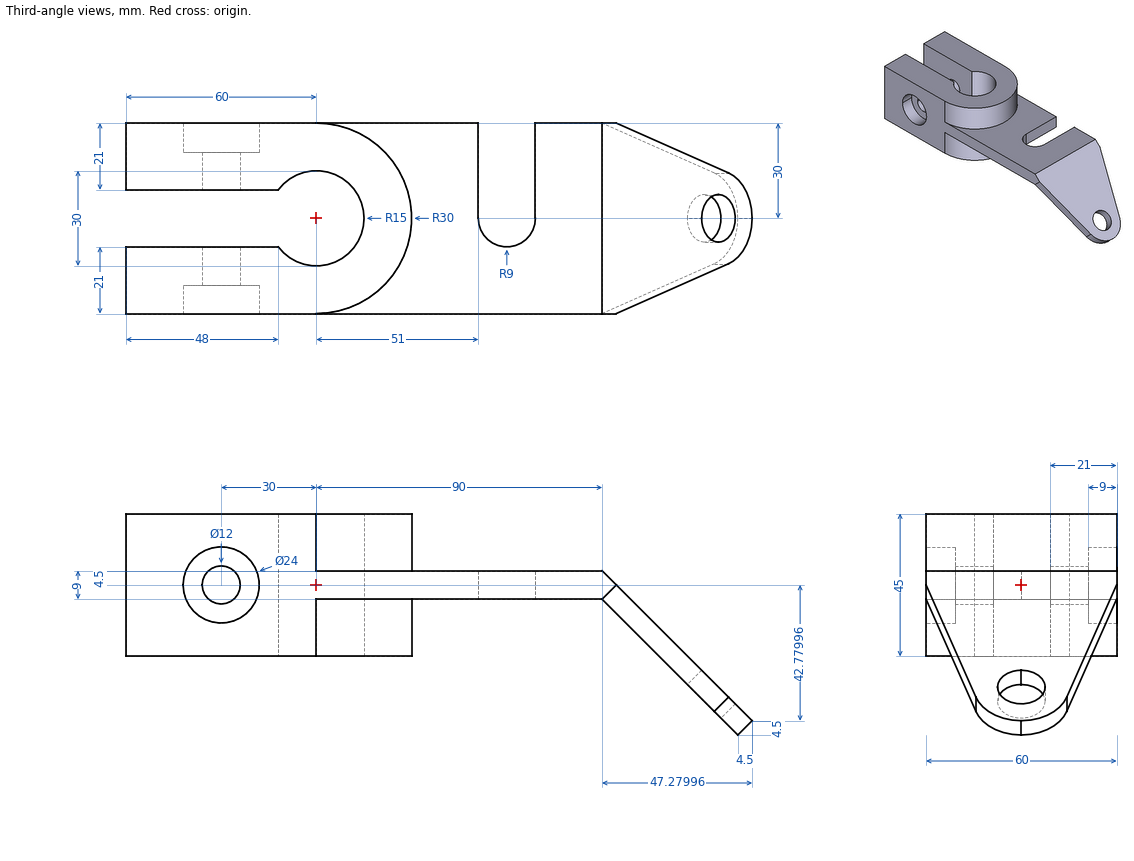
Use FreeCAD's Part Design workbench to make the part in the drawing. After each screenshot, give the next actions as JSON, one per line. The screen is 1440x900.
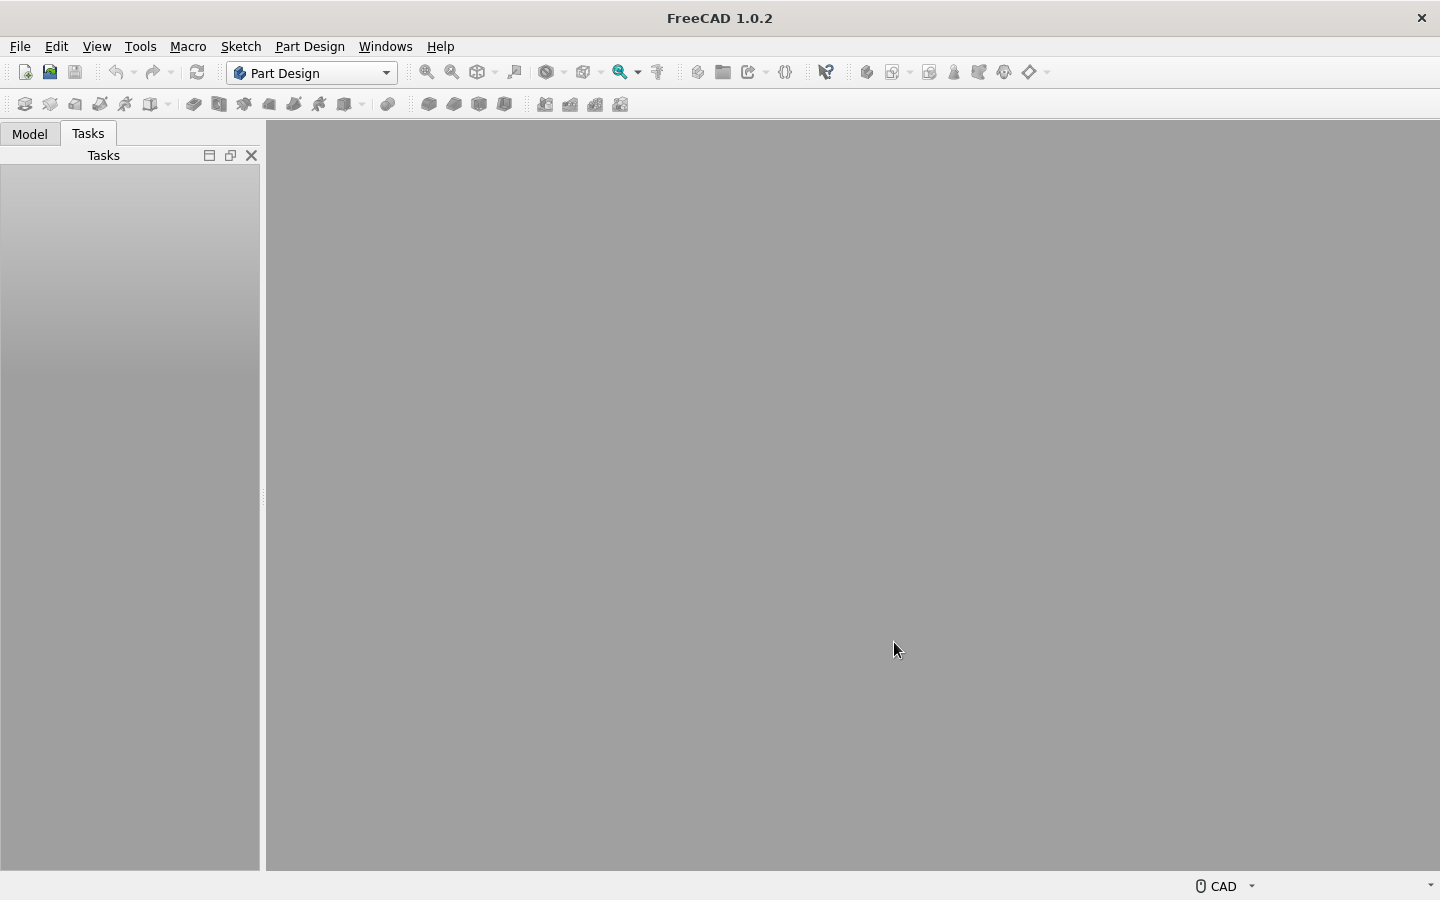
{"action": "left_click", "coordinate": [25, 72]}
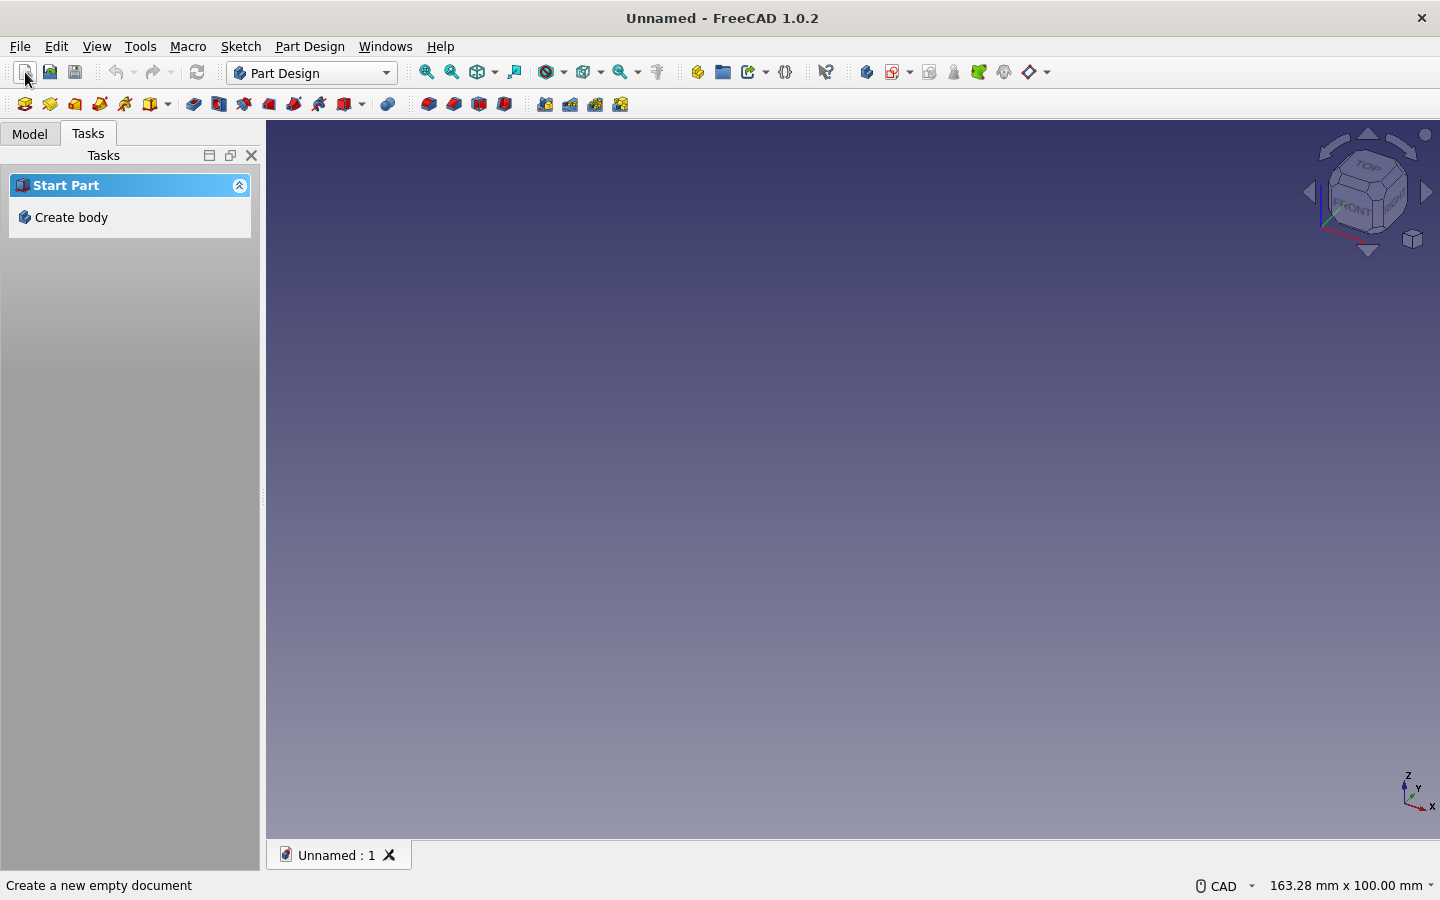
{"action": "left_click", "coordinate": [892, 72]}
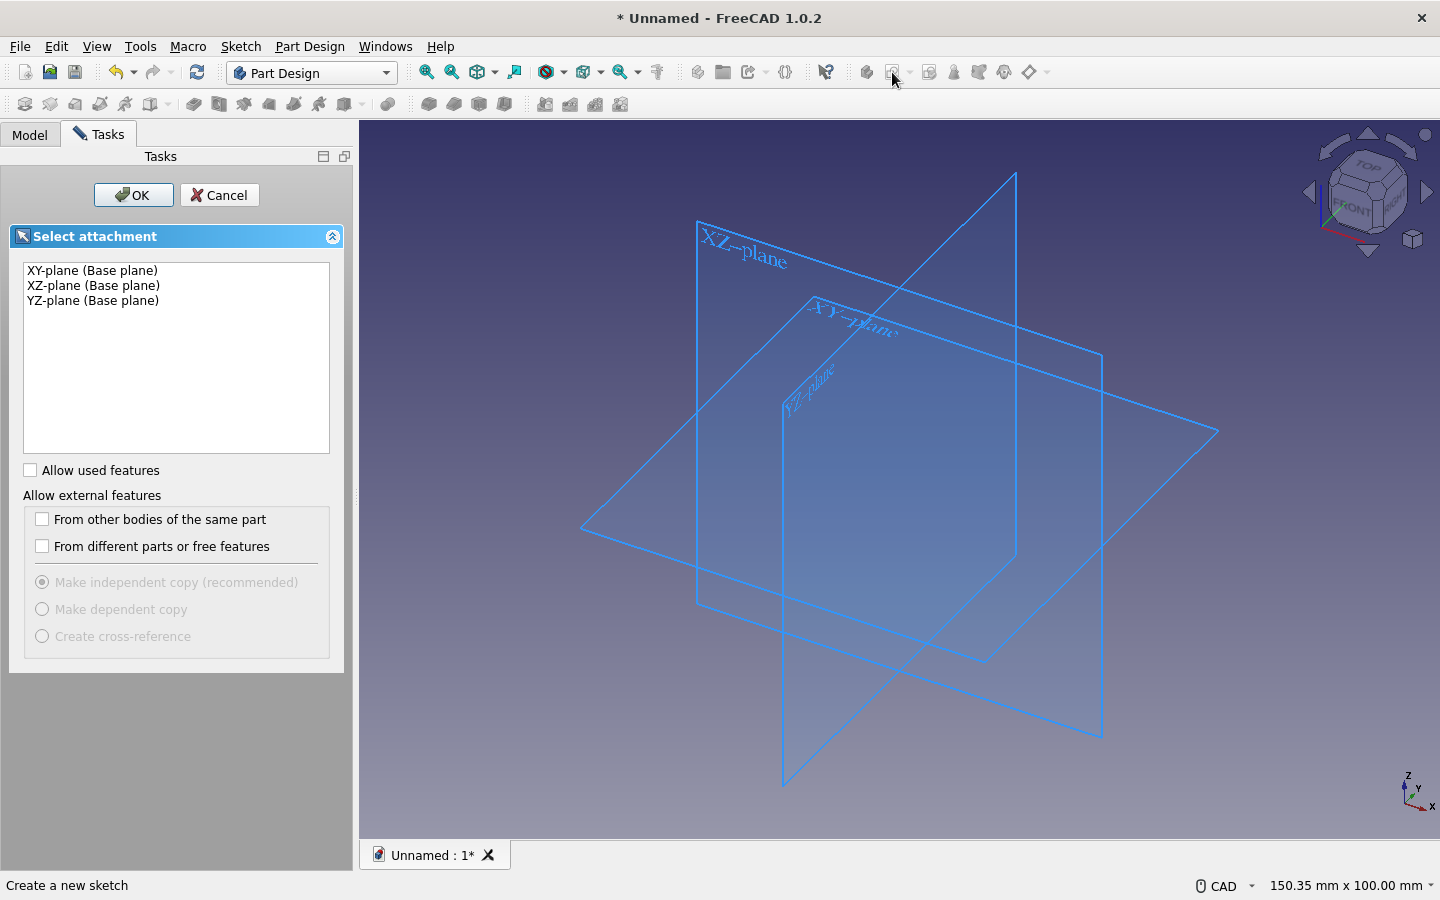
{"action": "left_click", "coordinate": [84, 270]}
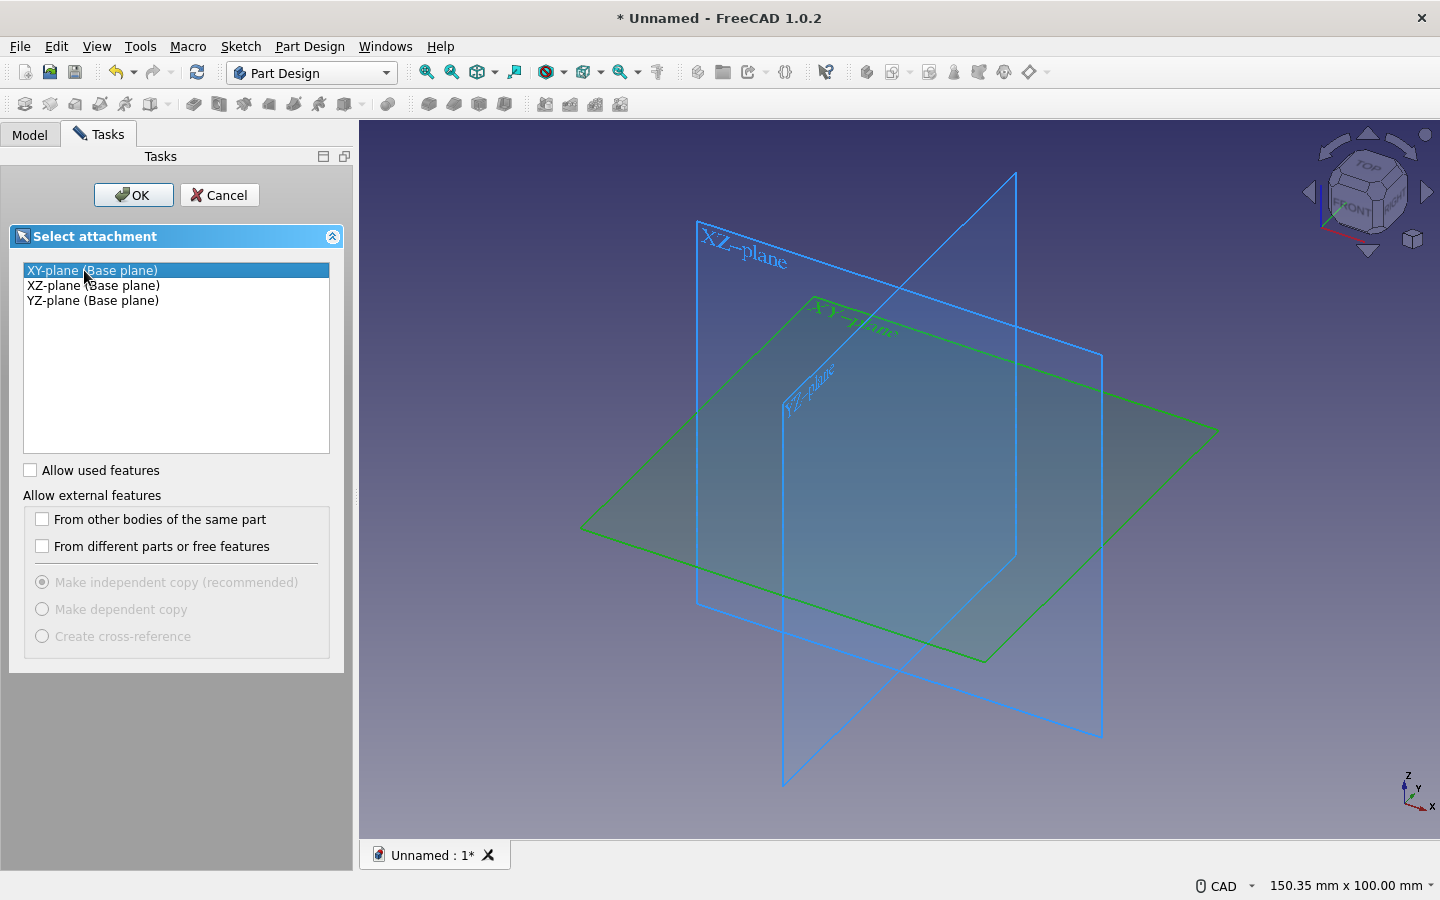
{"action": "left_click", "coordinate": [134, 195]}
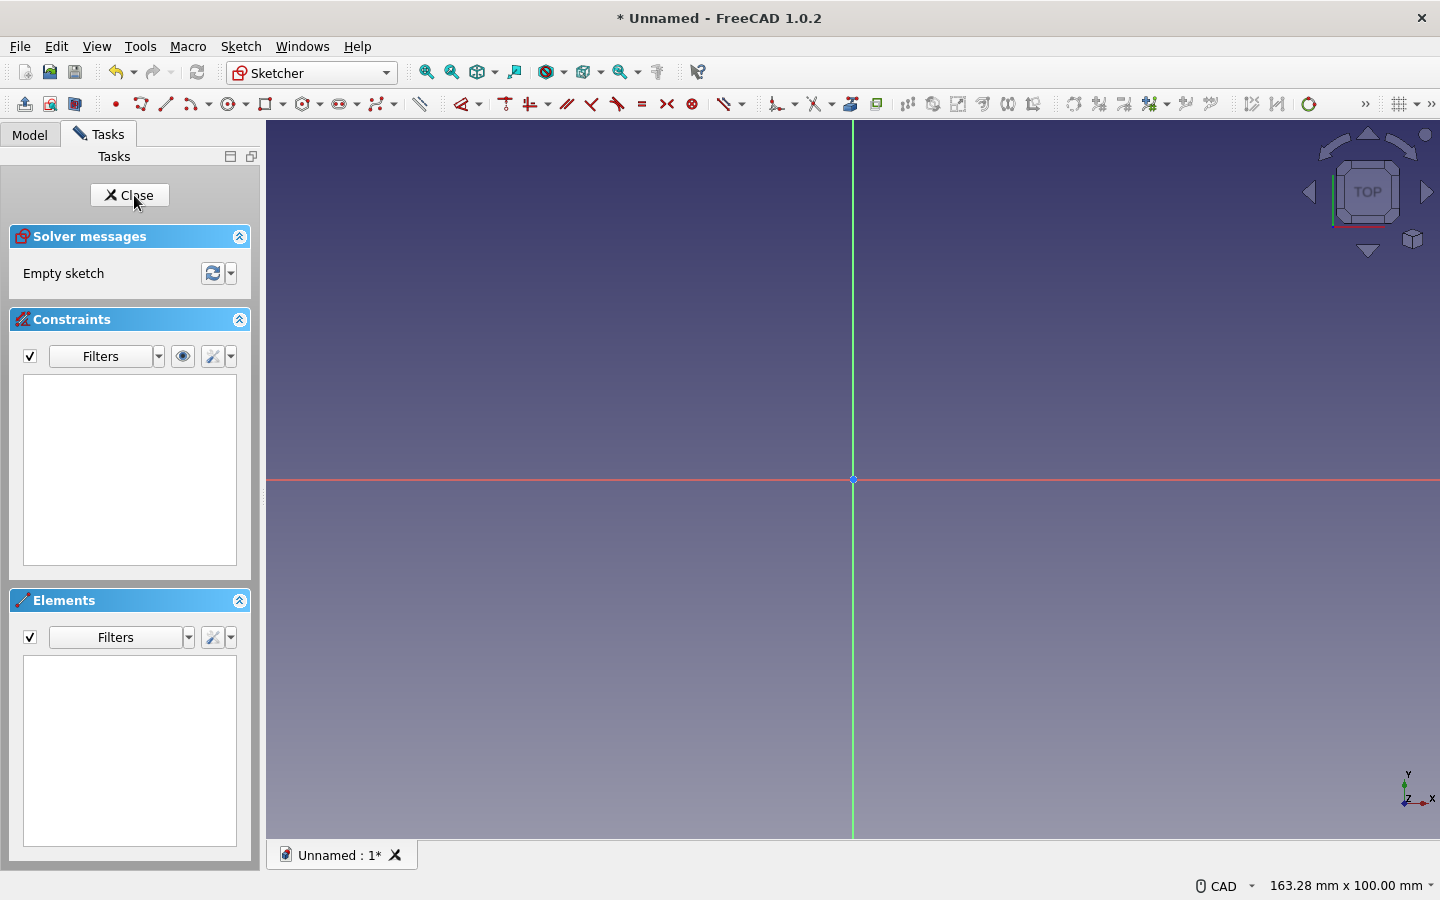
{"action": "left_click", "coordinate": [141, 104]}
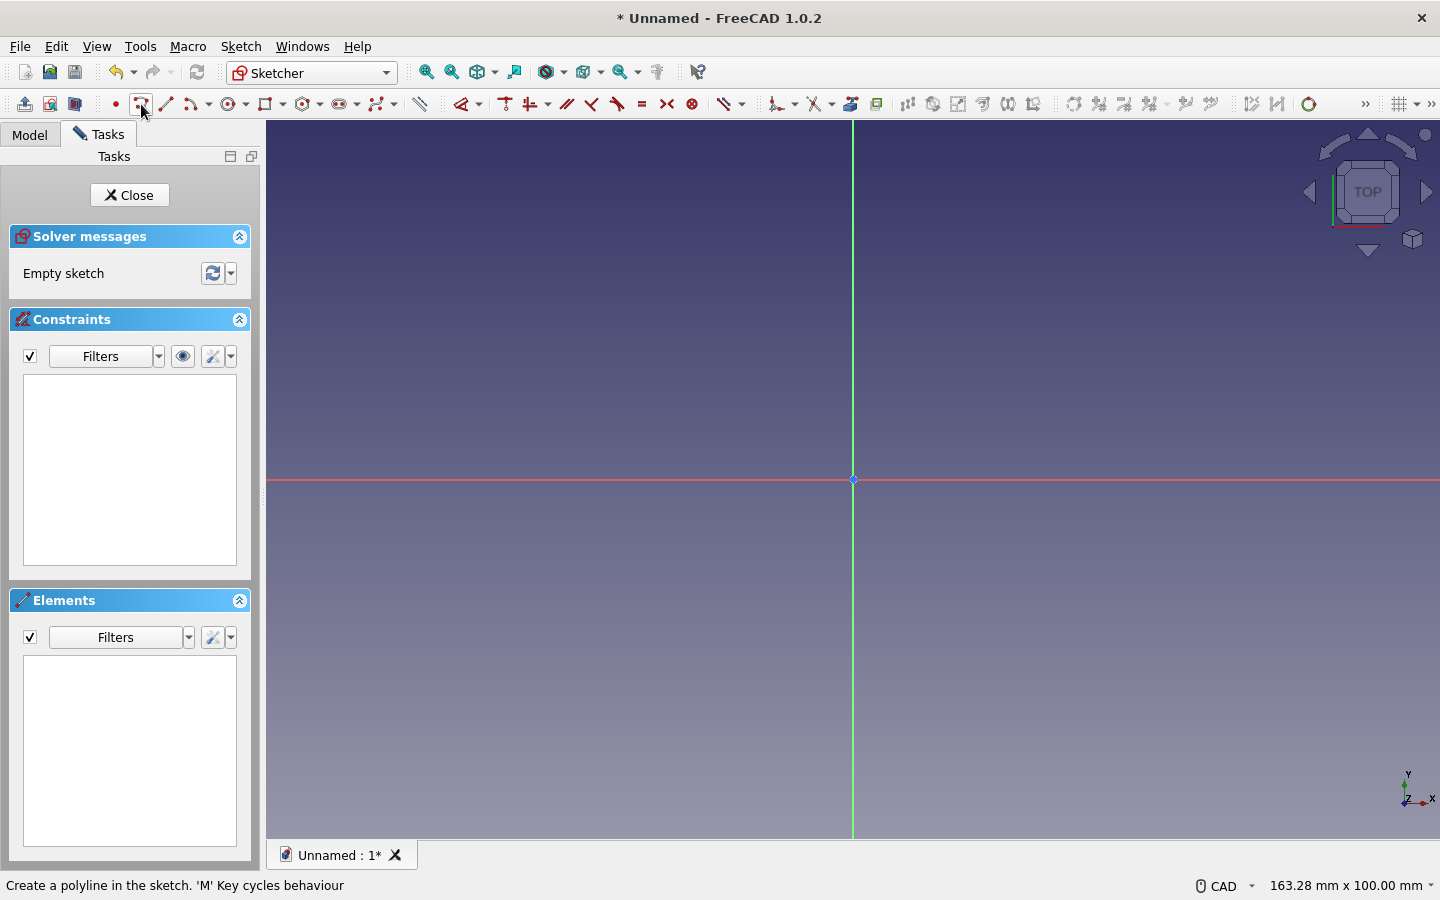
{"action": "left_click", "coordinate": [853, 264]}
{"action": "left_click", "coordinate": [422, 264]}
{"action": "left_click", "coordinate": [422, 415]}
{"action": "left_click", "coordinate": [767, 415]}
{"action": "right_click", "coordinate": [767, 415]}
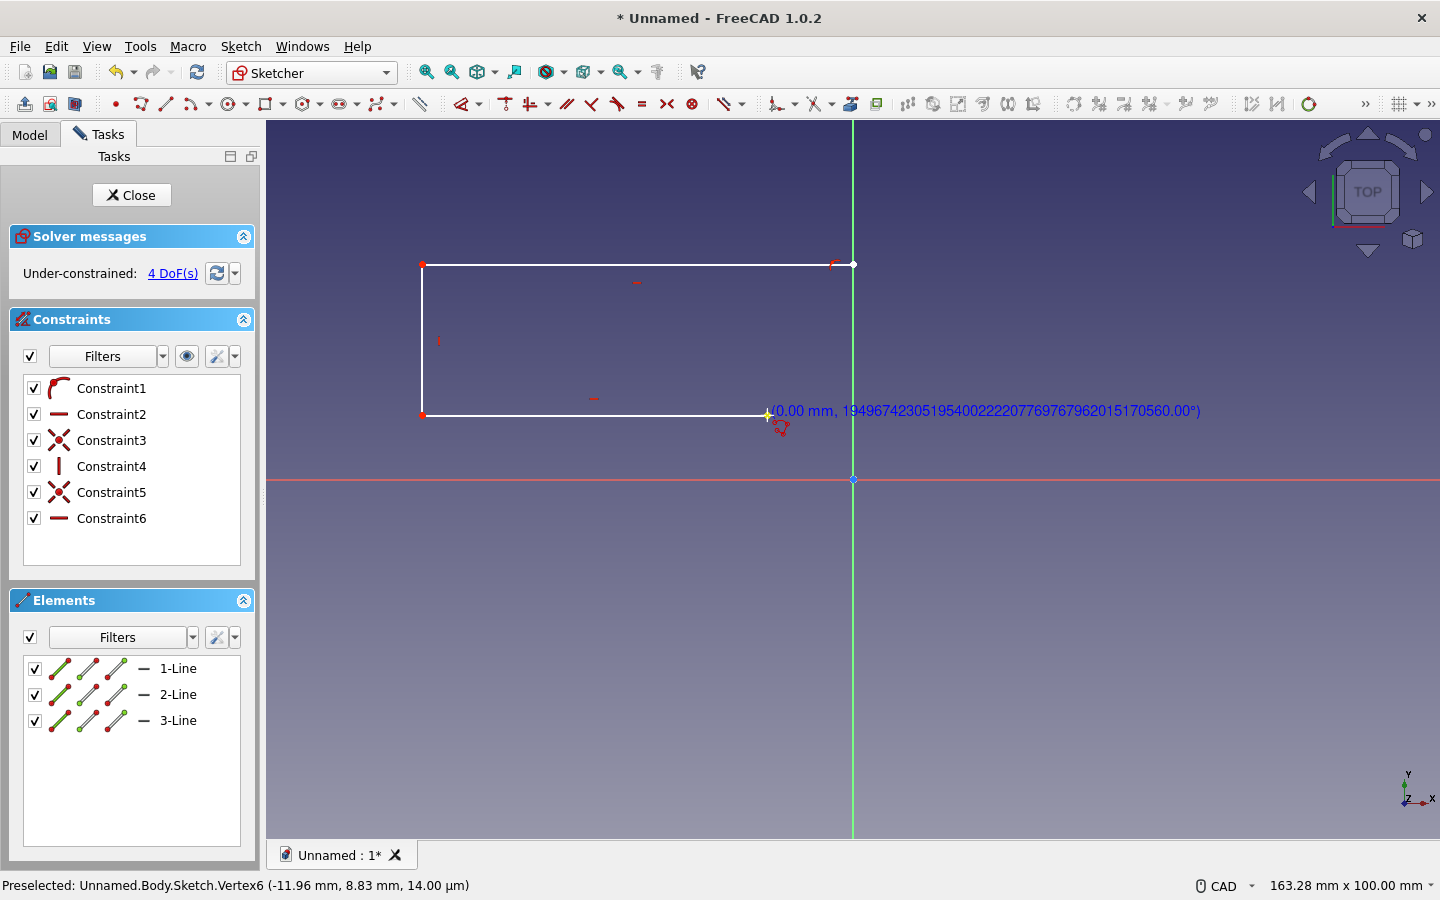
{"action": "left_click", "coordinate": [767, 544]}
{"action": "left_click", "coordinate": [422, 544]}
{"action": "left_click", "coordinate": [422, 695]}
{"action": "left_click", "coordinate": [853, 695]}
{"action": "right_click", "coordinate": [853, 695]}